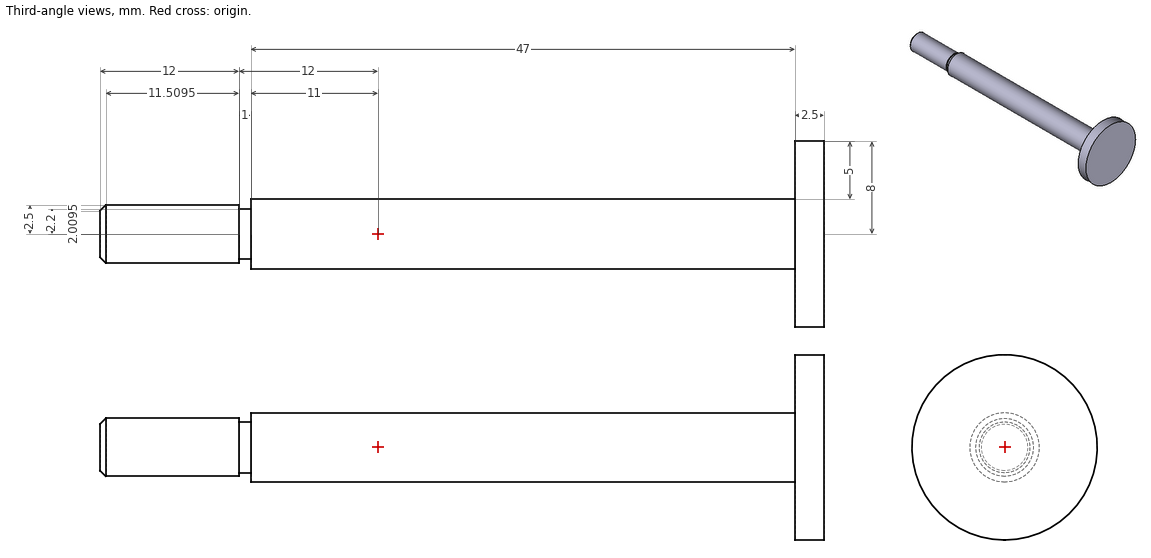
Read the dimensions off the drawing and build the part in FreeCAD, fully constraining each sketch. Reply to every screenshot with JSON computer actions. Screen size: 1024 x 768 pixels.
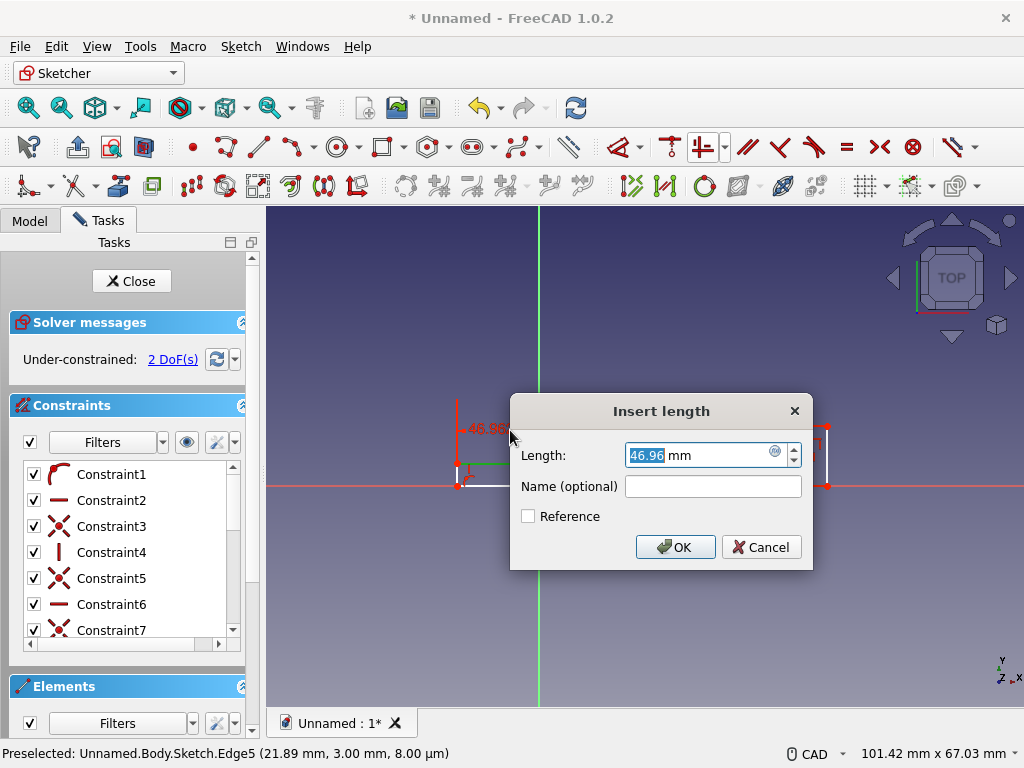
{"action": "type", "text": "47"}
{"action": "key", "text": "Return"}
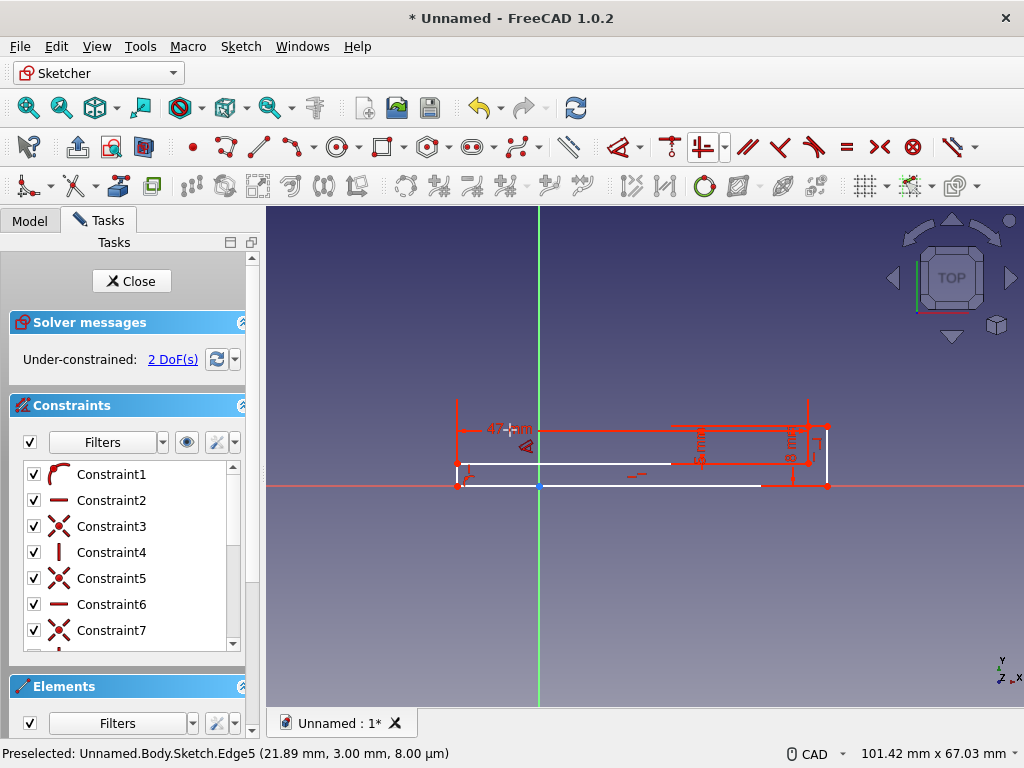
{"action": "scroll", "coordinate": [818, 426], "scroll_direction": "up", "scroll_amount": 4}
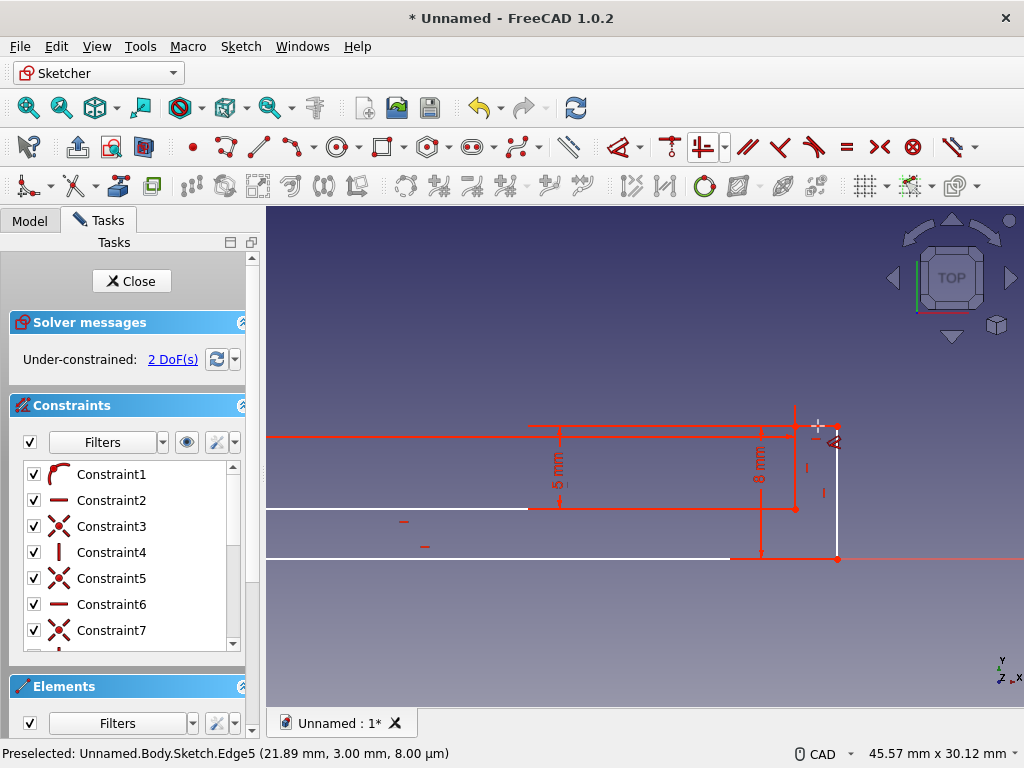
{"action": "left_click", "coordinate": [816, 426]}
{"action": "left_click", "coordinate": [816, 392]}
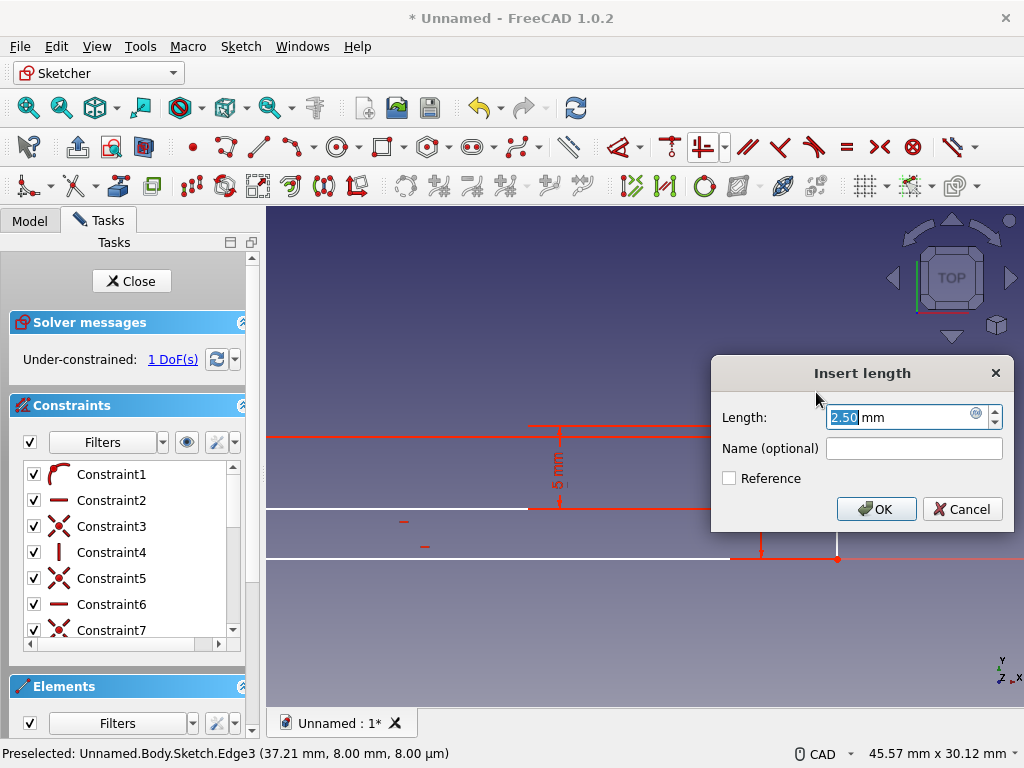
{"action": "type", "text": "2.5"}
{"action": "key", "text": "Return"}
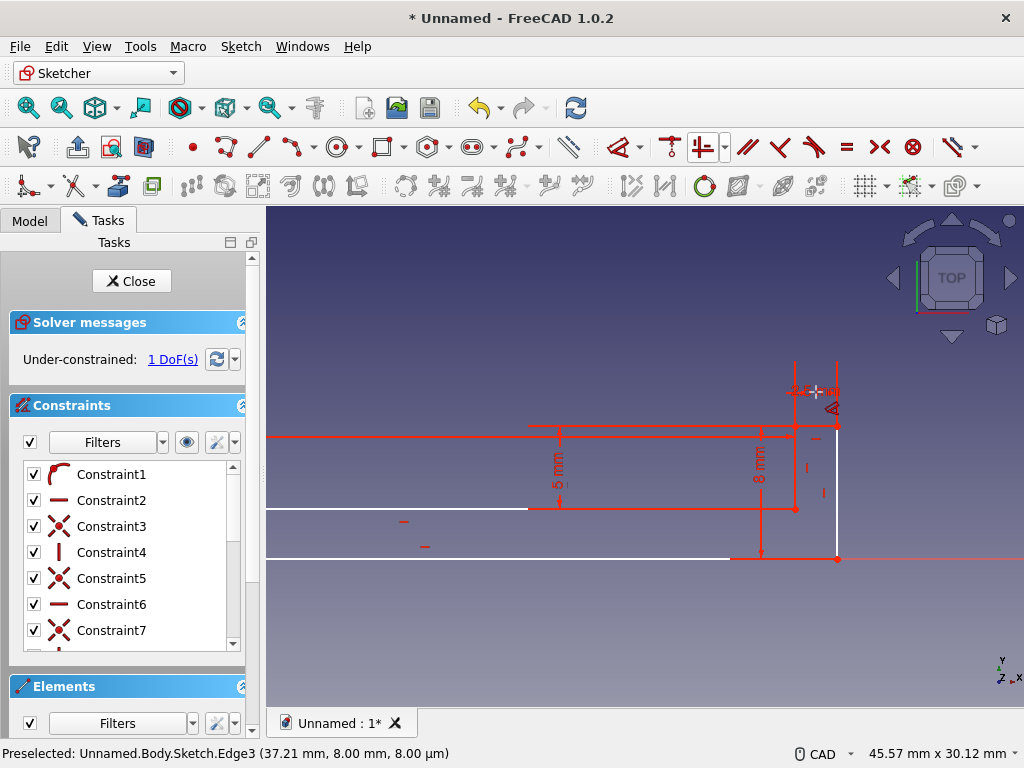
{"action": "scroll", "coordinate": [700, 427], "scroll_direction": "down", "scroll_amount": 4}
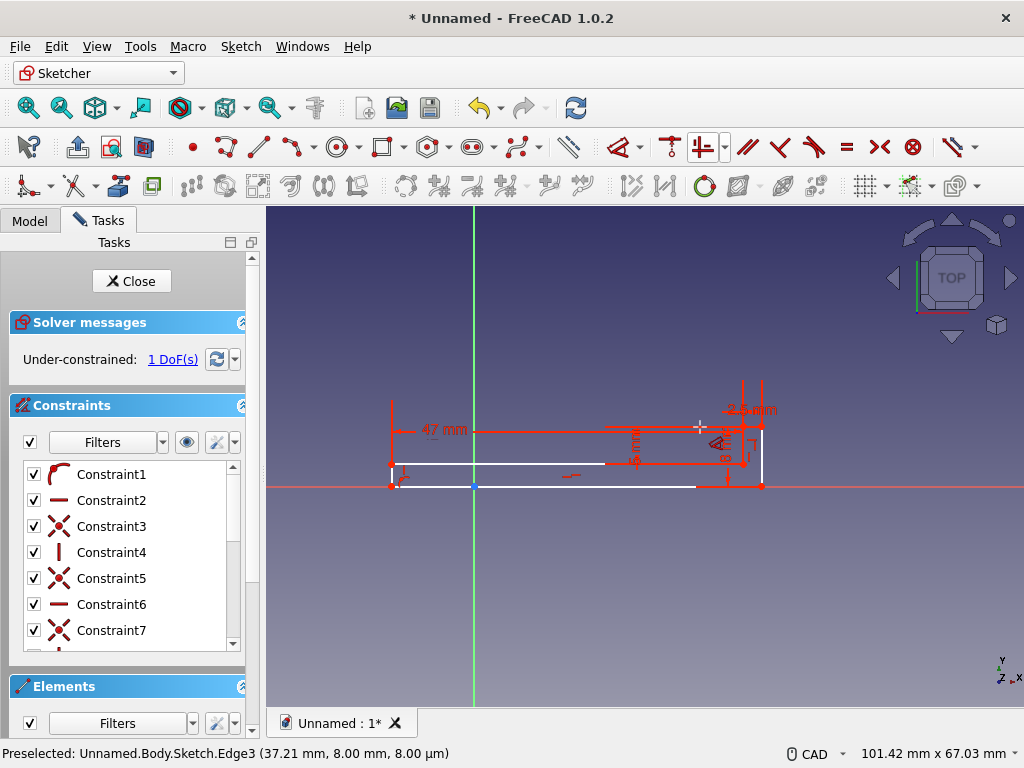
{"action": "left_click", "coordinate": [392, 487]}
{"action": "left_click", "coordinate": [433, 521]}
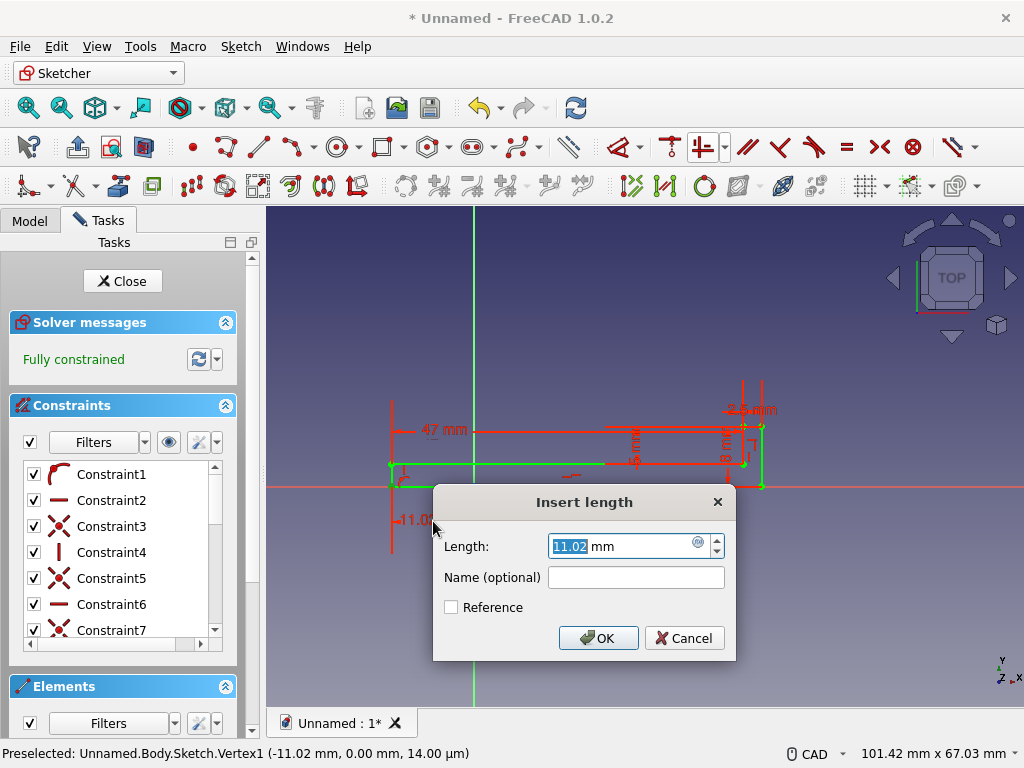
{"action": "type", "text": "11"}
{"action": "key", "text": "Return"}
{"action": "key", "text": "Escape"}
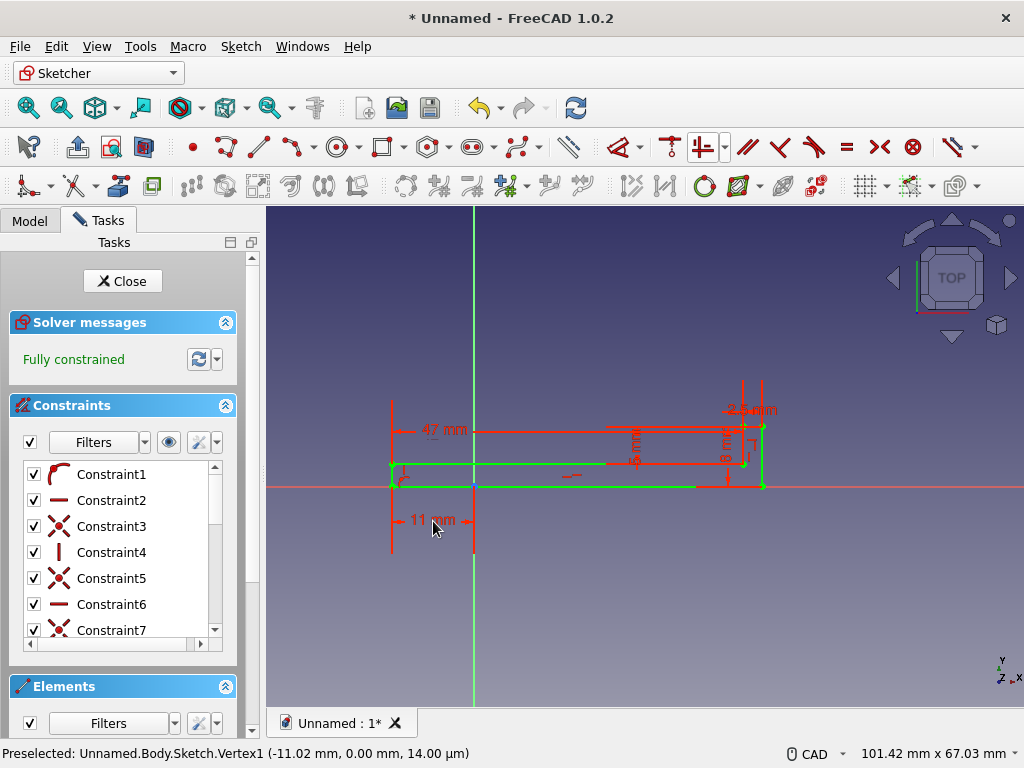
{"action": "left_click", "coordinate": [123, 281]}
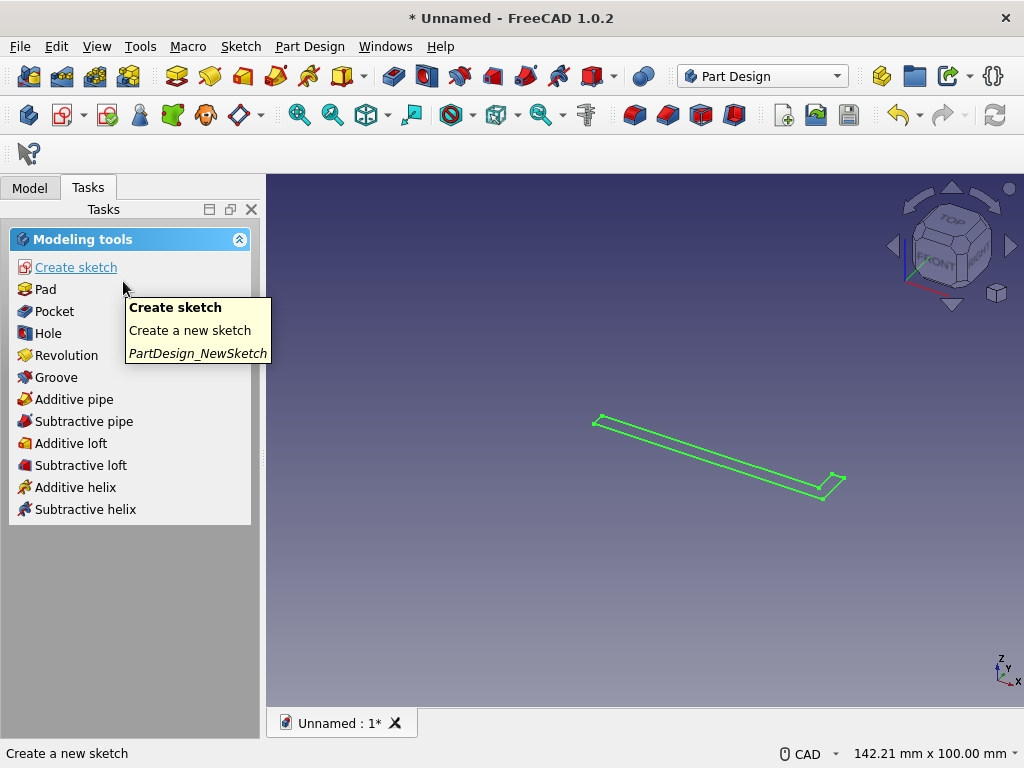
{"action": "left_click", "coordinate": [210, 76]}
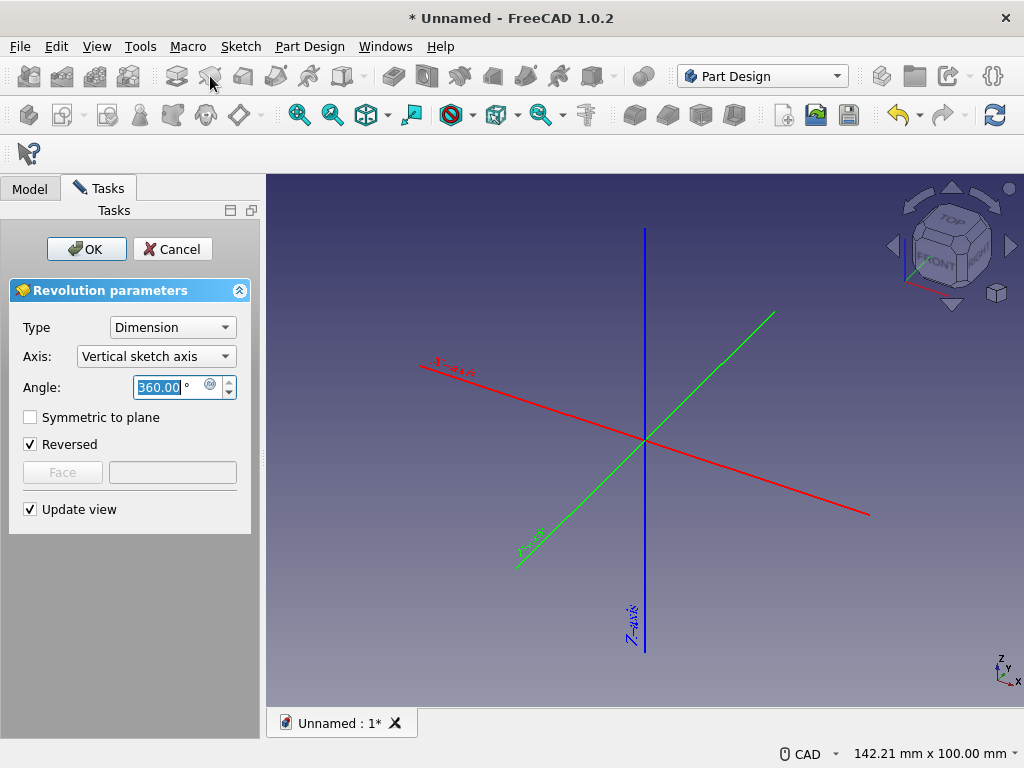
{"action": "left_click", "coordinate": [157, 356]}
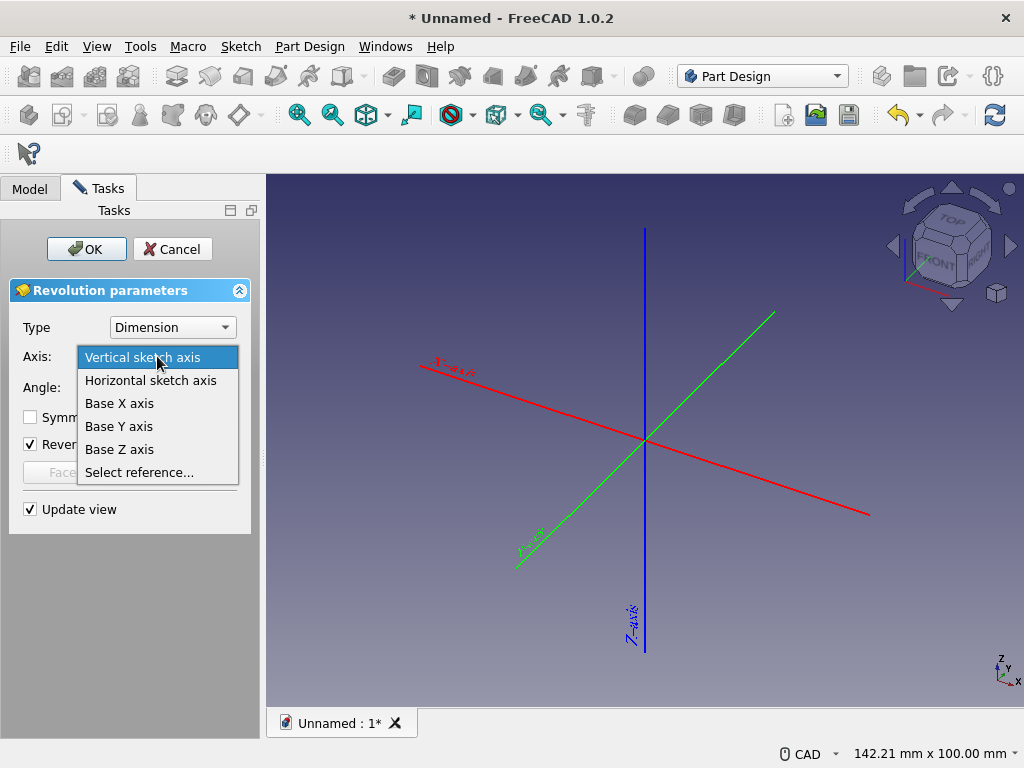
{"action": "left_click", "coordinate": [156, 380]}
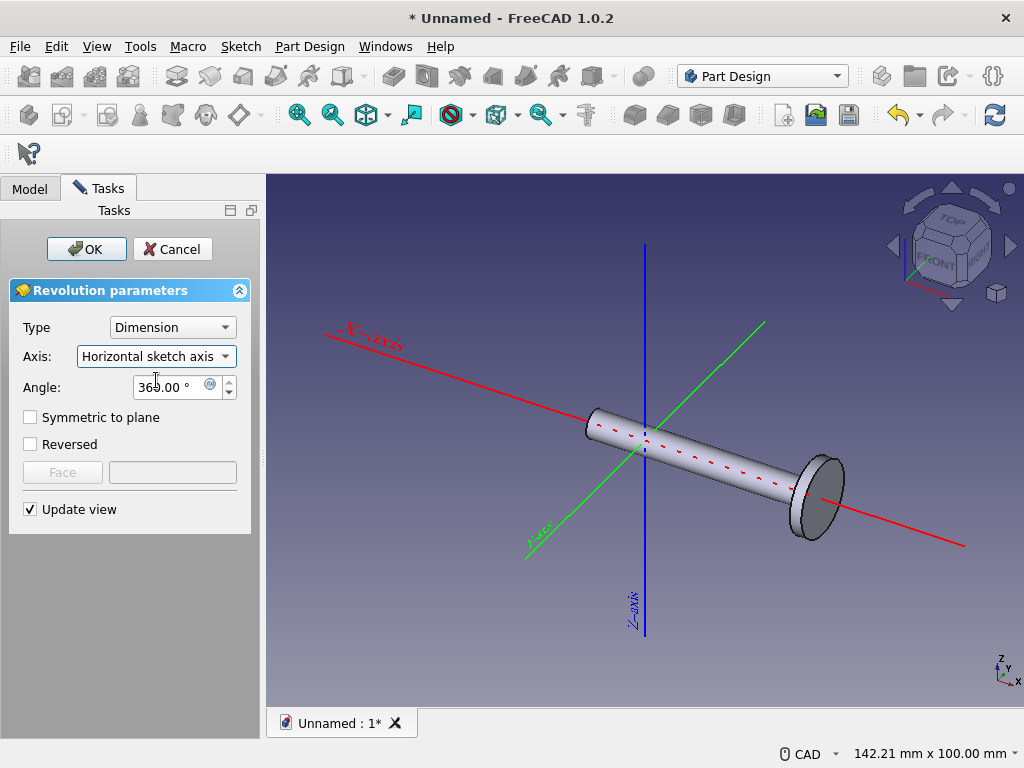
{"action": "left_click", "coordinate": [87, 249]}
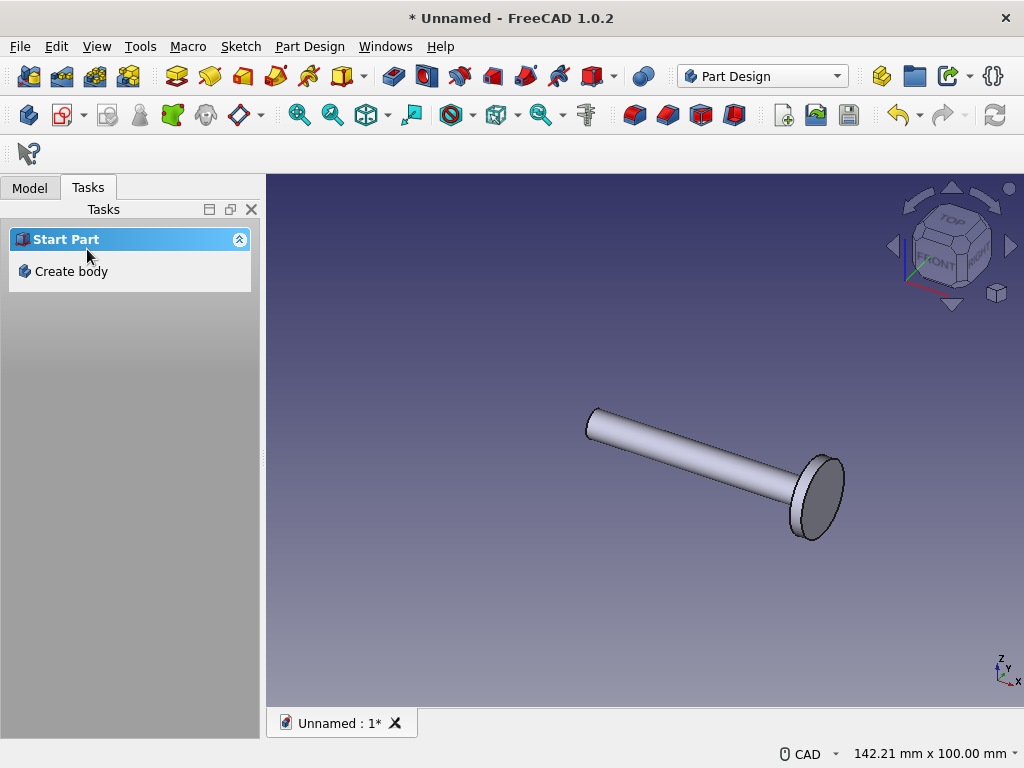
{"action": "left_click", "coordinate": [300, 116]}